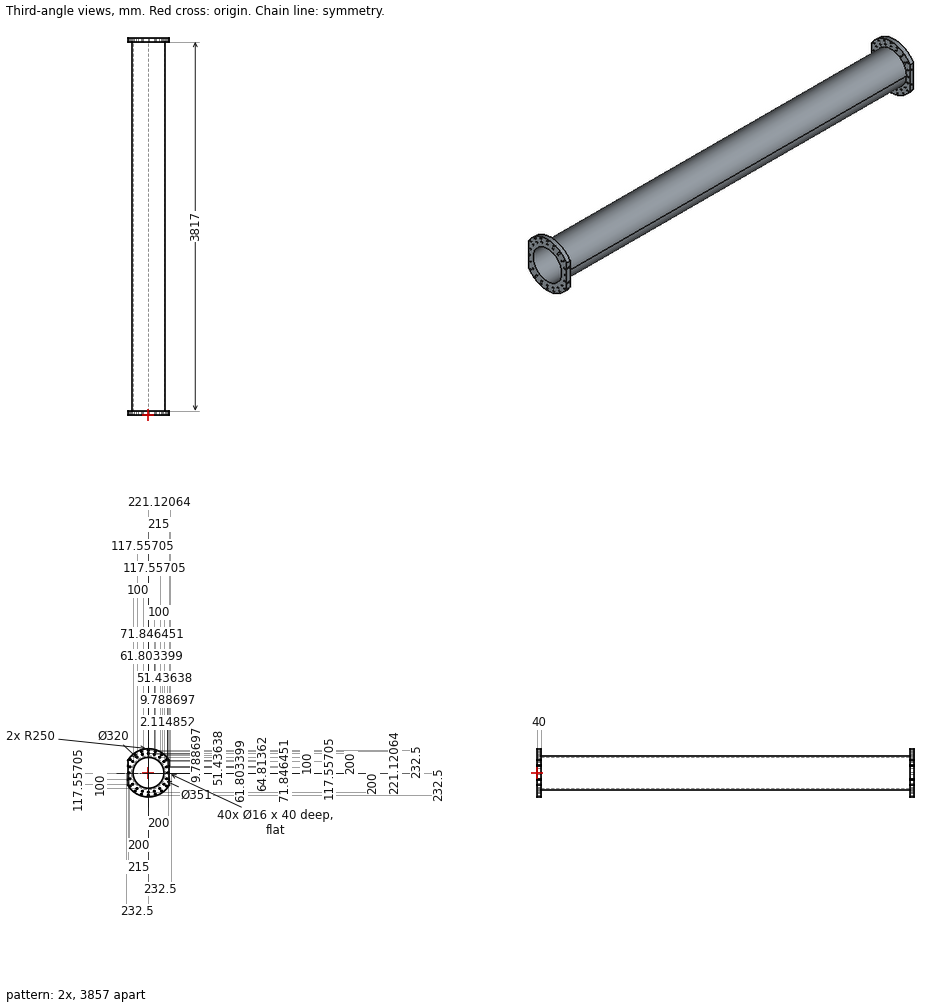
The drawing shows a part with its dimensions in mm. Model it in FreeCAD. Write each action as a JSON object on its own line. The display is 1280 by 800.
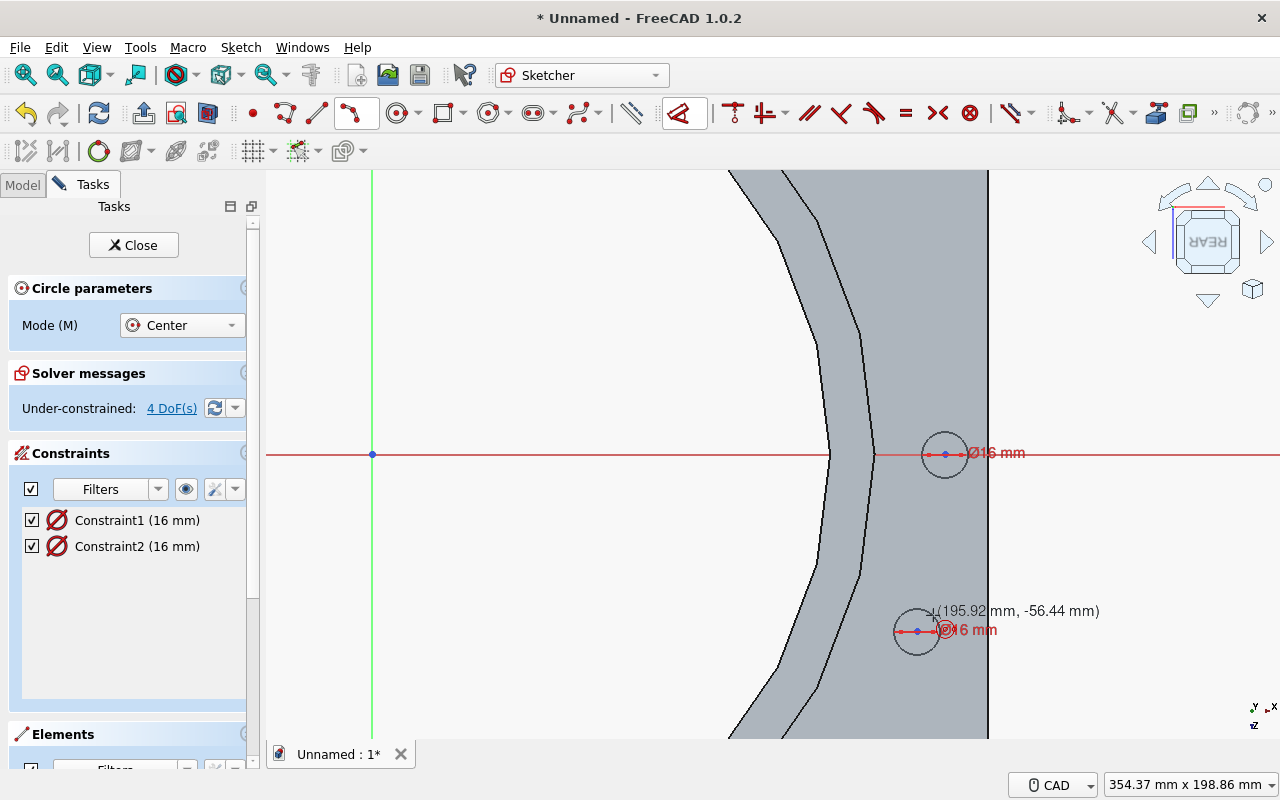
{"action": "scroll", "coordinate": [813, 455], "scroll_direction": "down", "scroll_amount": 7}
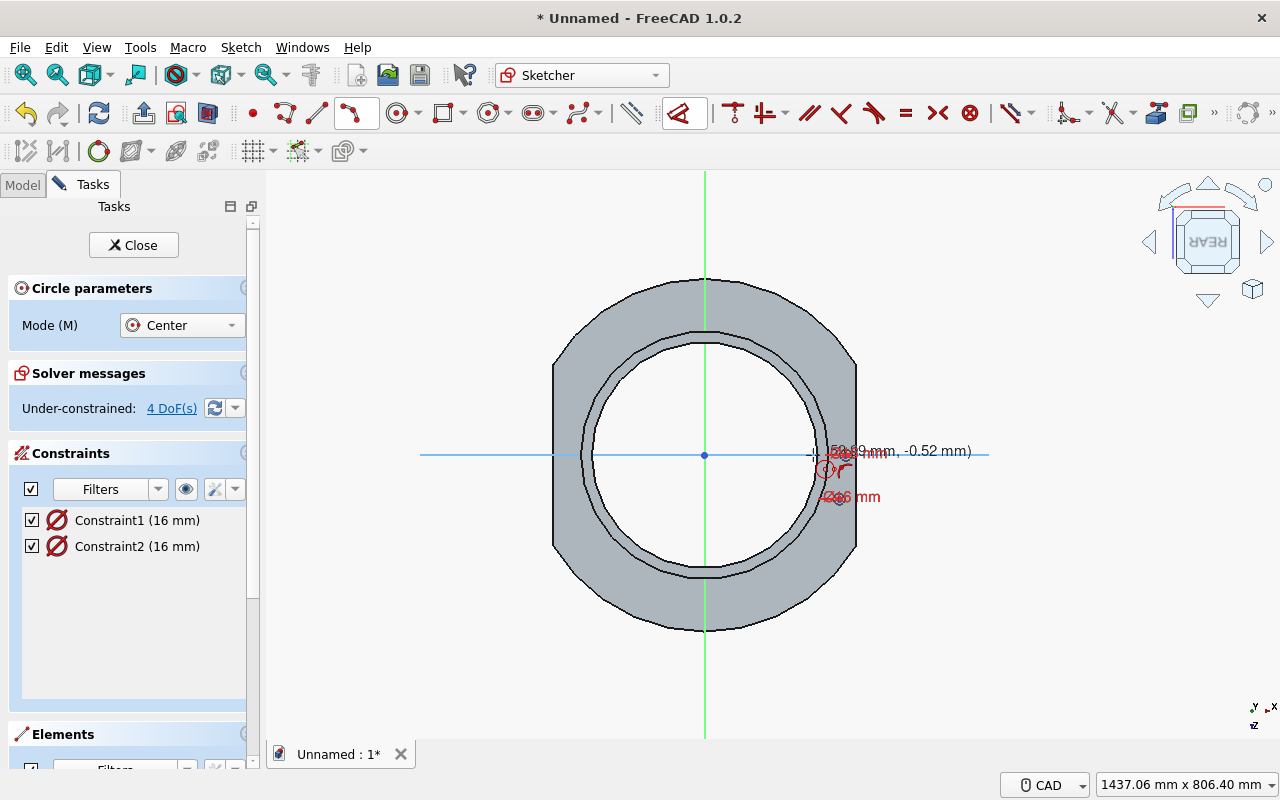
{"action": "scroll", "coordinate": [819, 538], "scroll_direction": "up", "scroll_amount": 7}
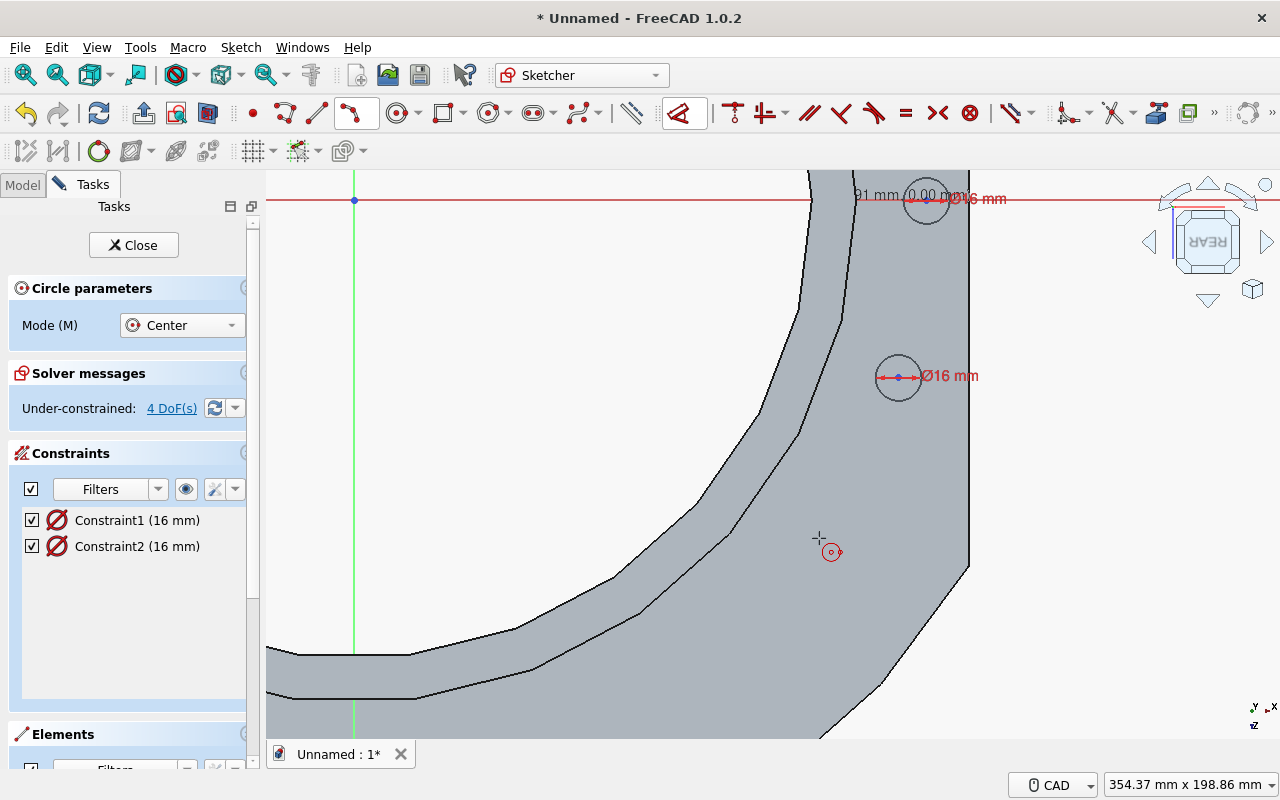
{"action": "left_click", "coordinate": [817, 537]}
{"action": "mouse_move", "coordinate": [833, 521]}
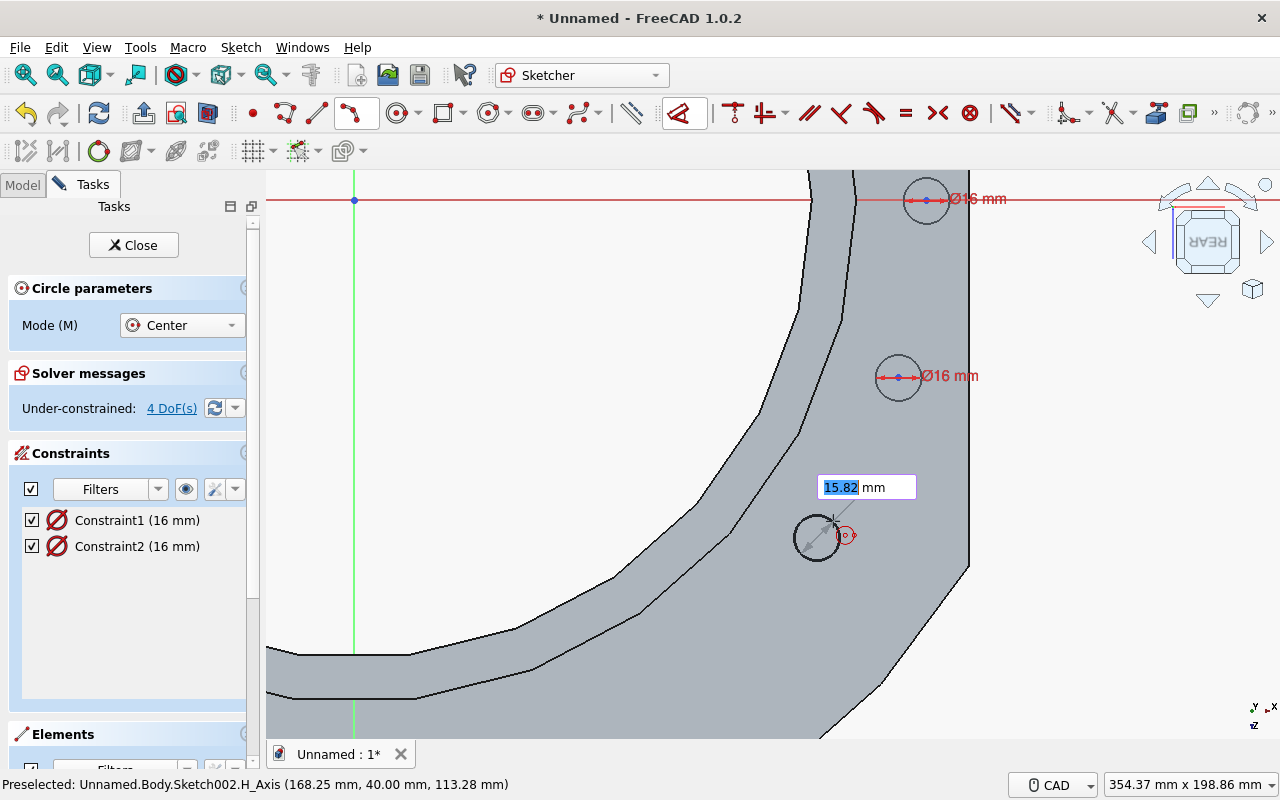
{"action": "type", "text": "16"}
{"action": "key", "text": "Return"}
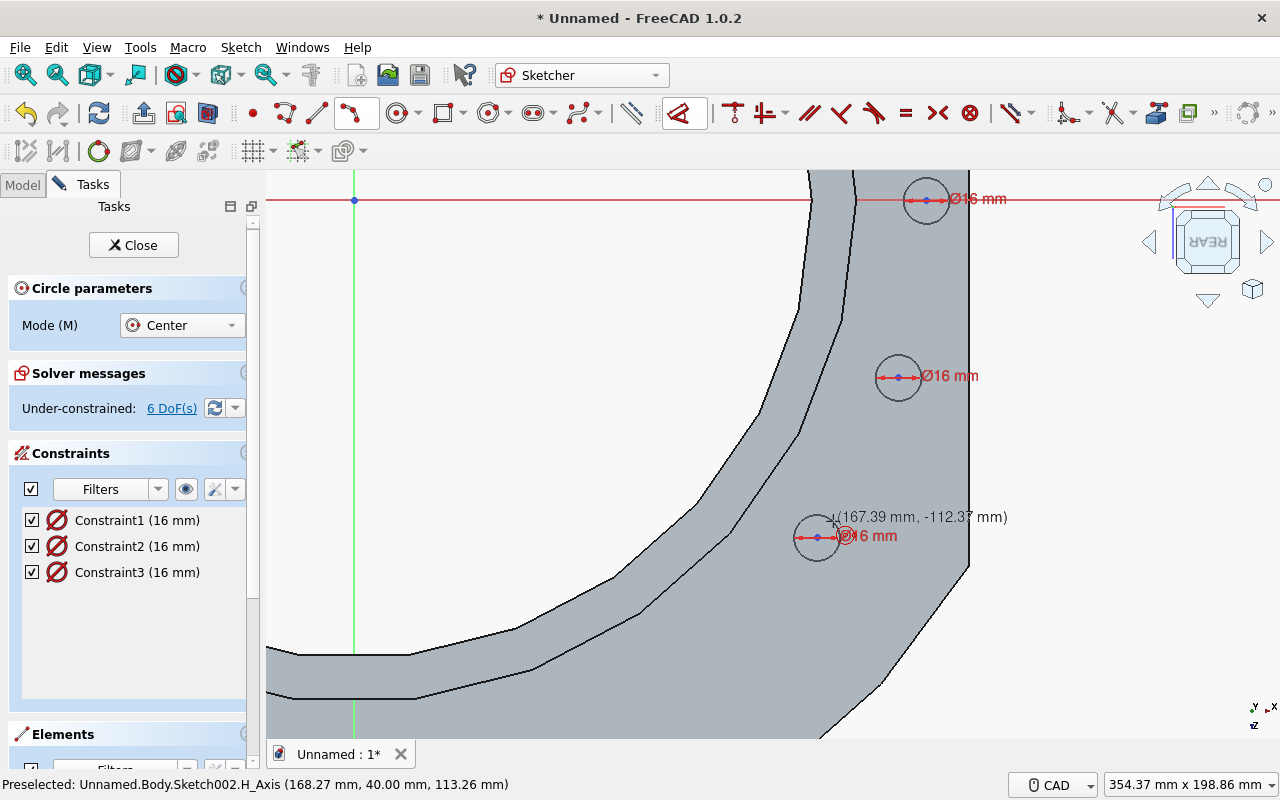
{"action": "left_click", "coordinate": [690, 663]}
{"action": "mouse_move", "coordinate": [707, 647]}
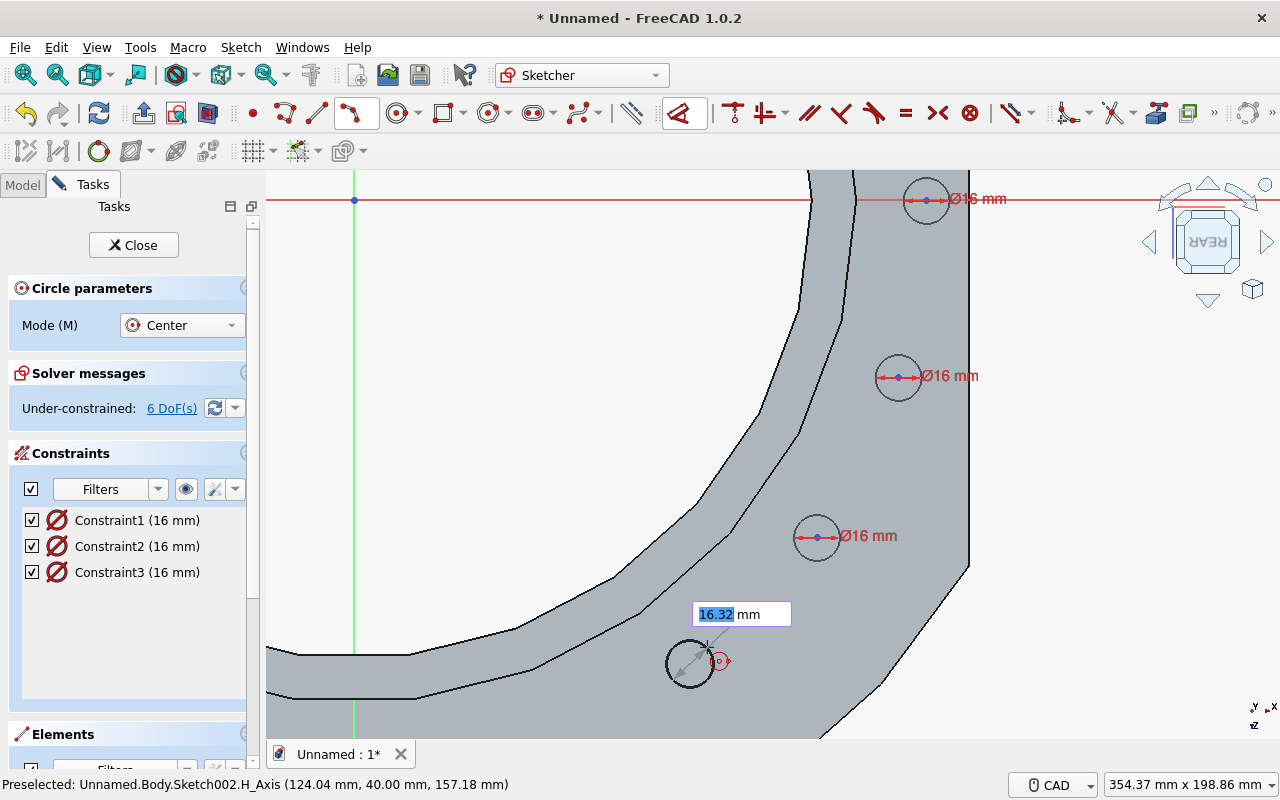
{"action": "type", "text": "16"}
{"action": "key", "text": "Return"}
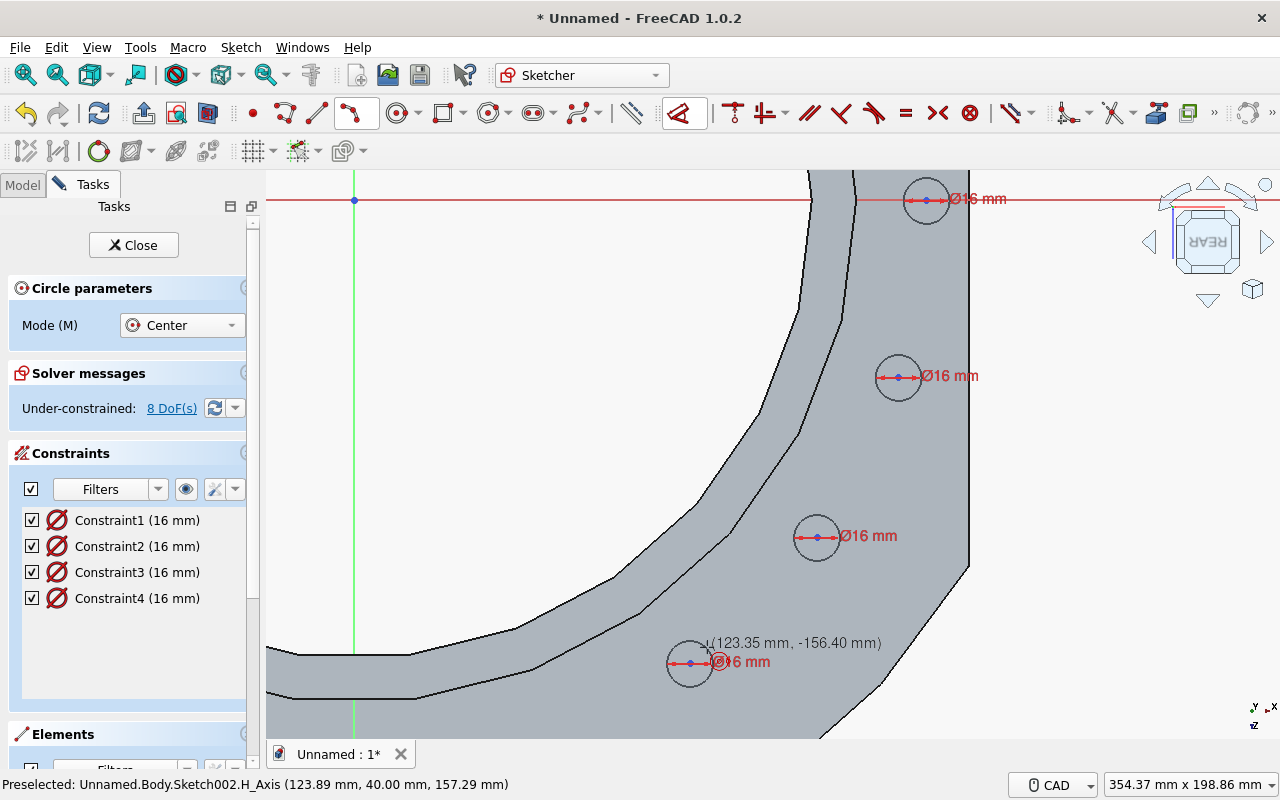
{"action": "scroll", "coordinate": [819, 538], "scroll_direction": "down", "scroll_amount": 7}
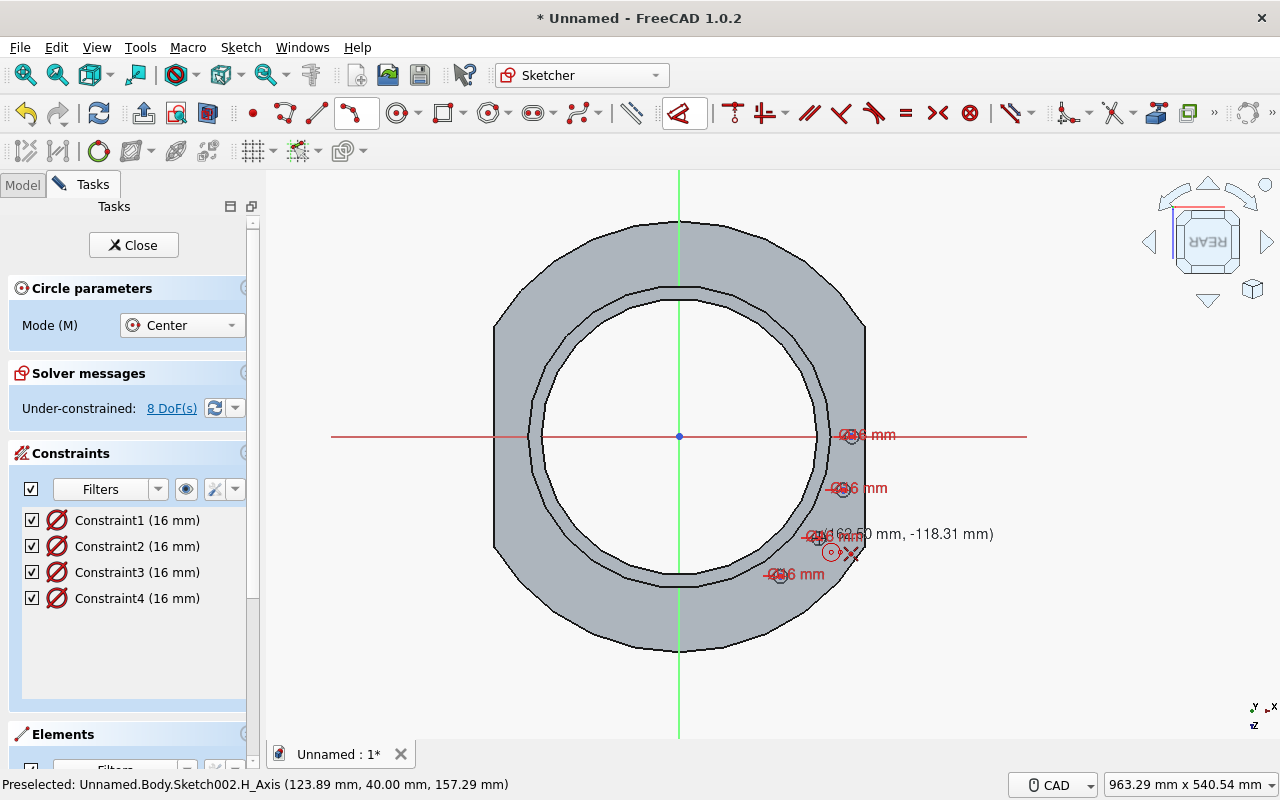
{"action": "scroll", "coordinate": [748, 589], "scroll_direction": "up", "scroll_amount": 7}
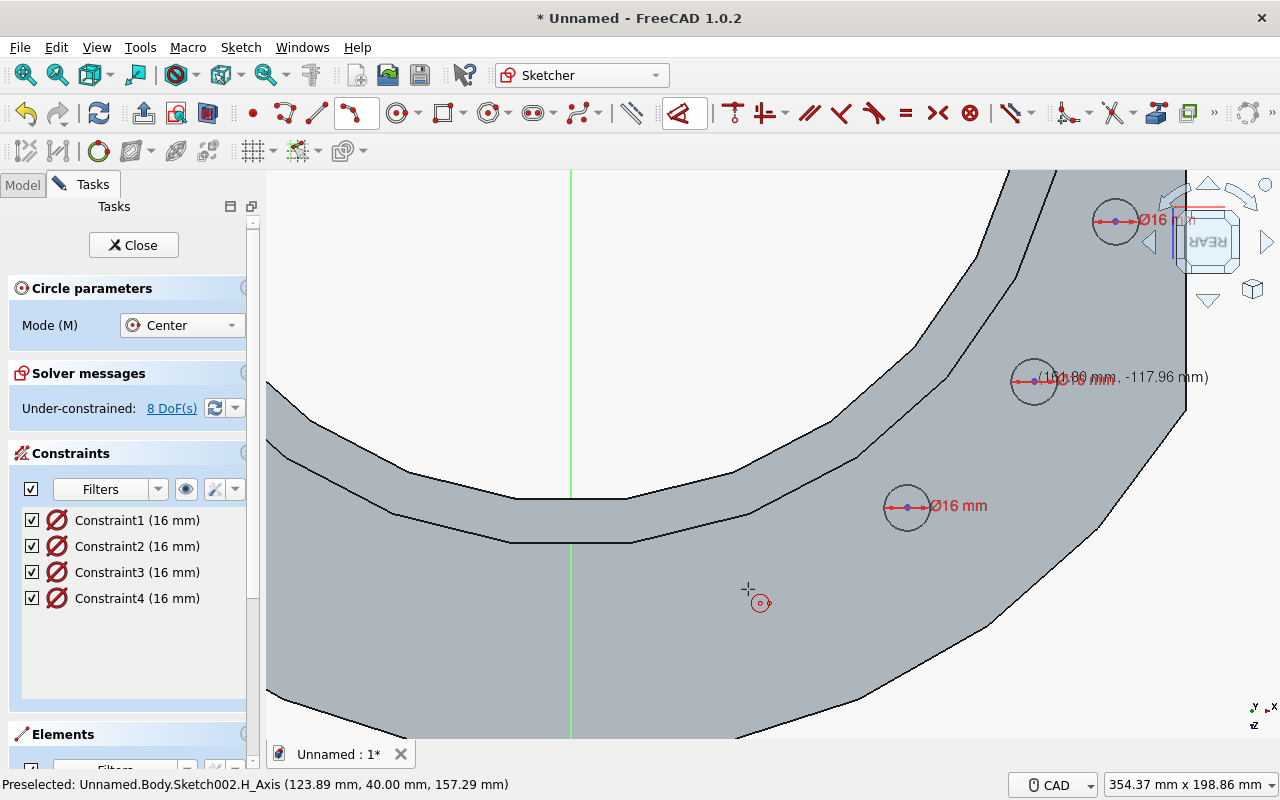
{"action": "left_click", "coordinate": [748, 589]}
{"action": "mouse_move", "coordinate": [764, 572]}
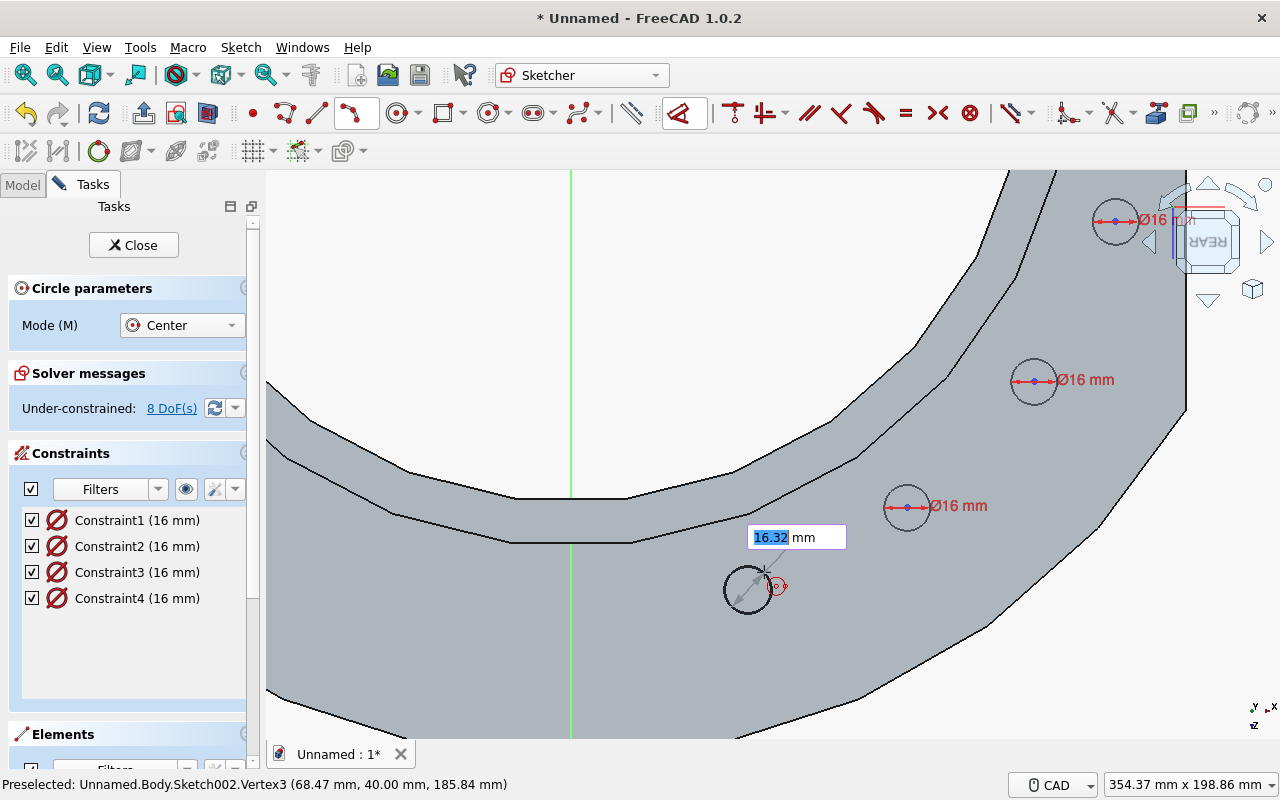
{"action": "type", "text": "16"}
{"action": "key", "text": "Return"}